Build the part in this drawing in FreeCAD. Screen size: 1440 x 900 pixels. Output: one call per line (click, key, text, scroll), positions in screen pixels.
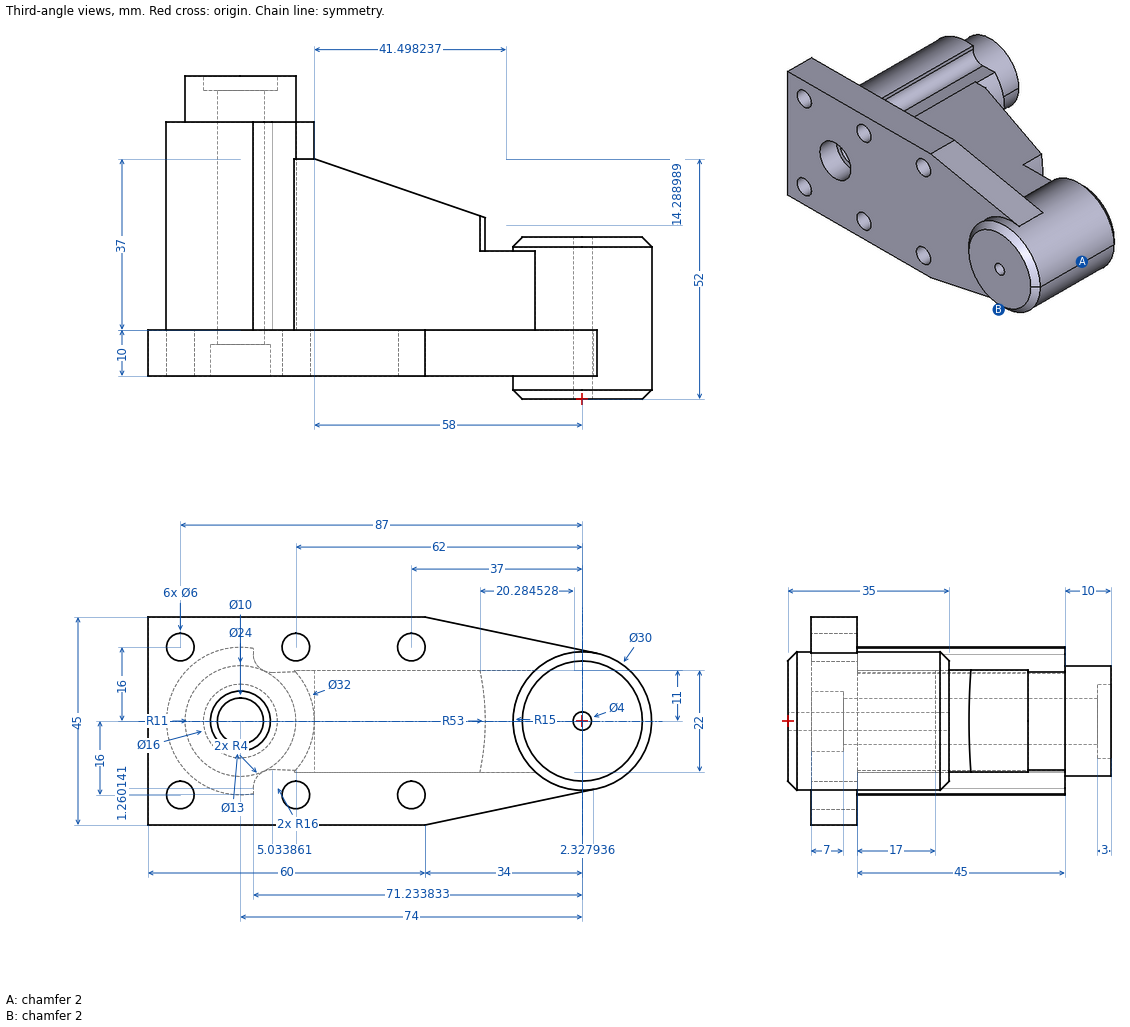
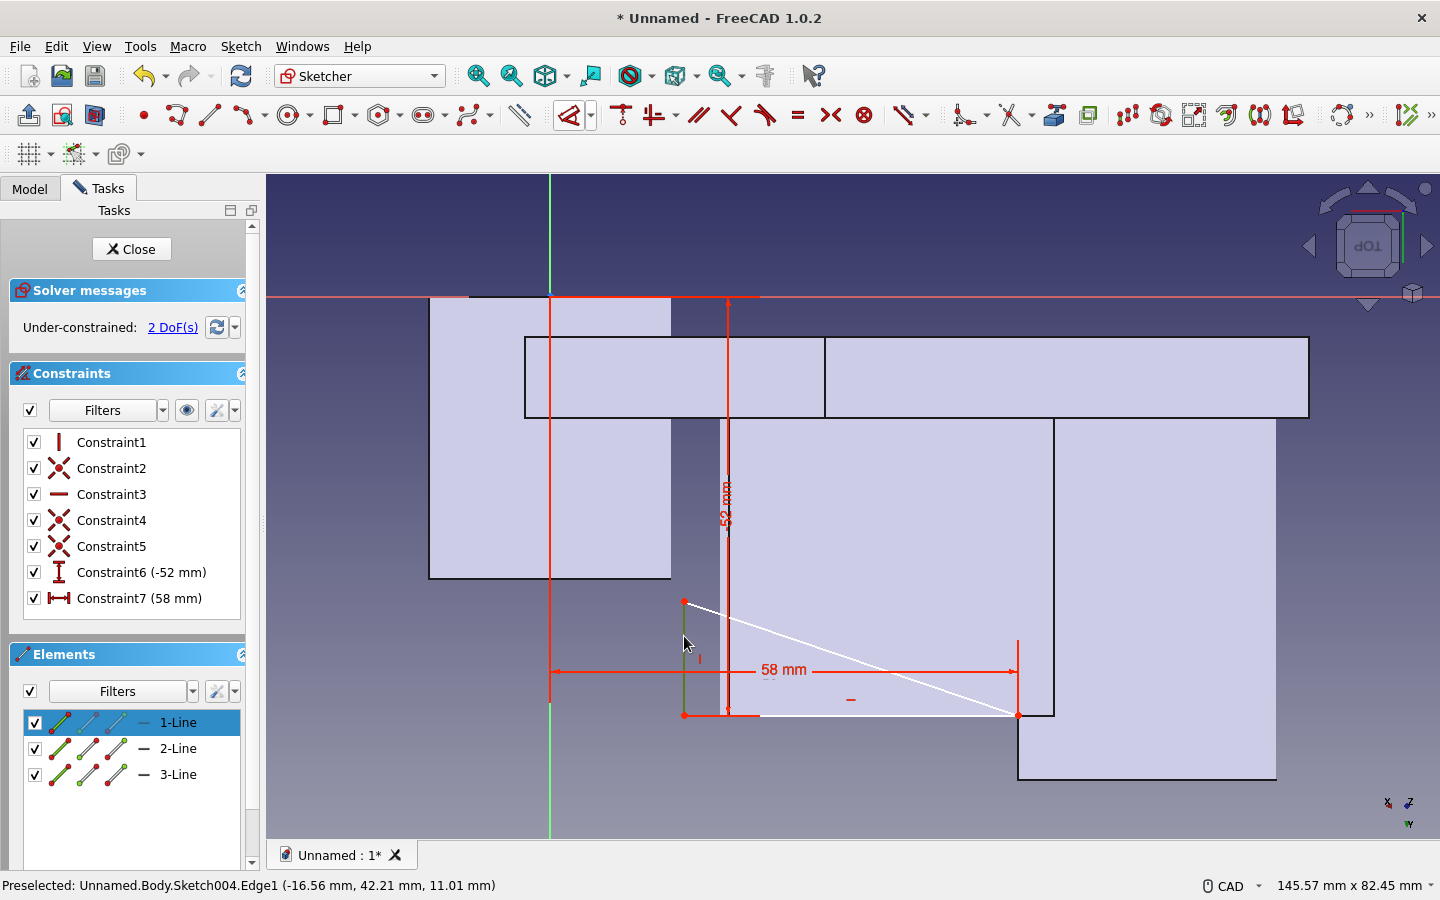
click(590, 116)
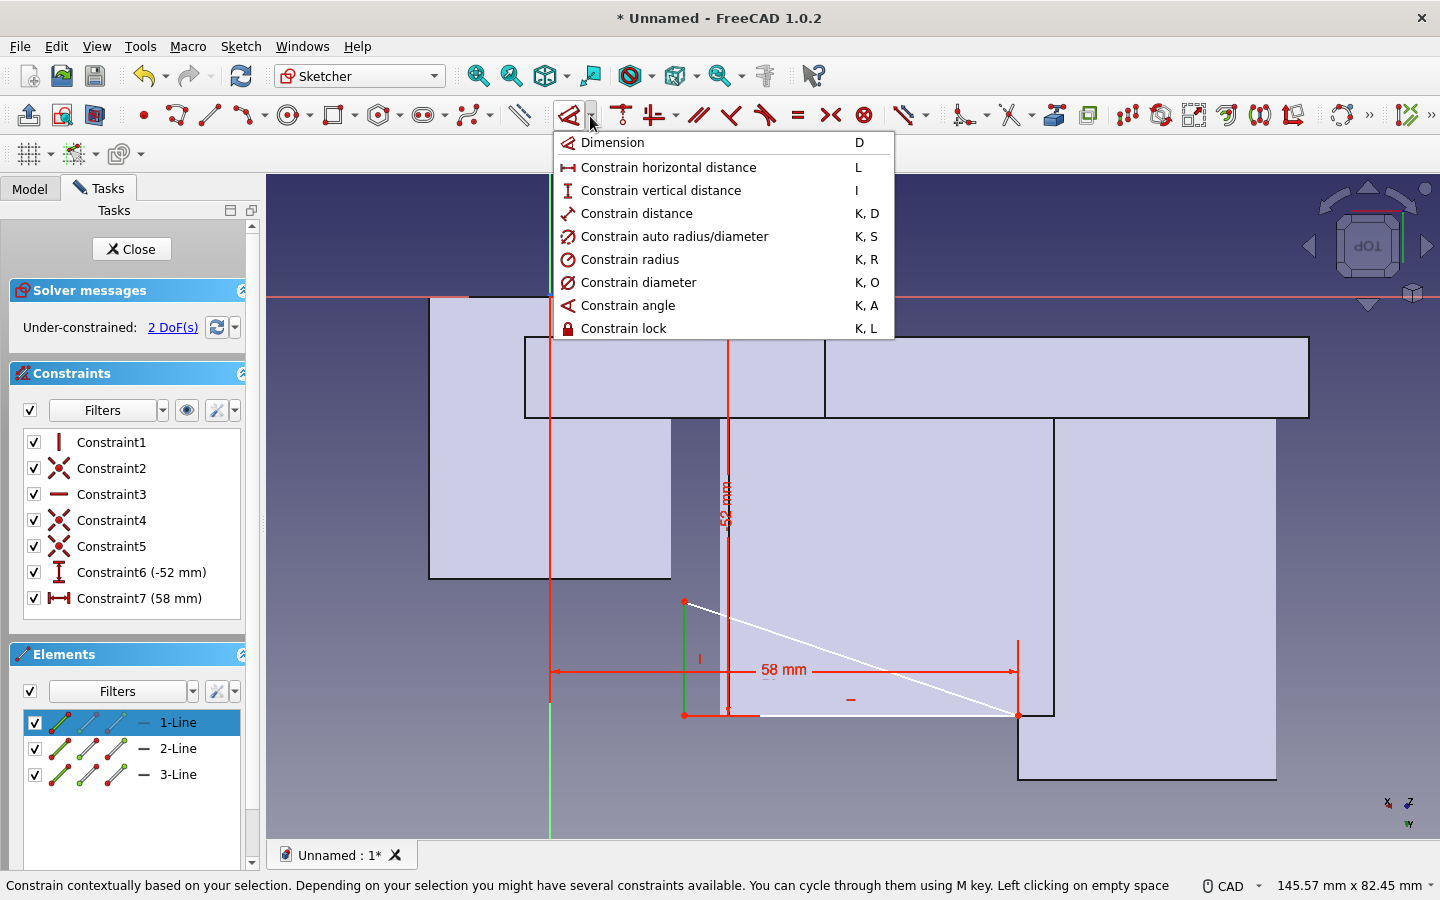
click(724, 190)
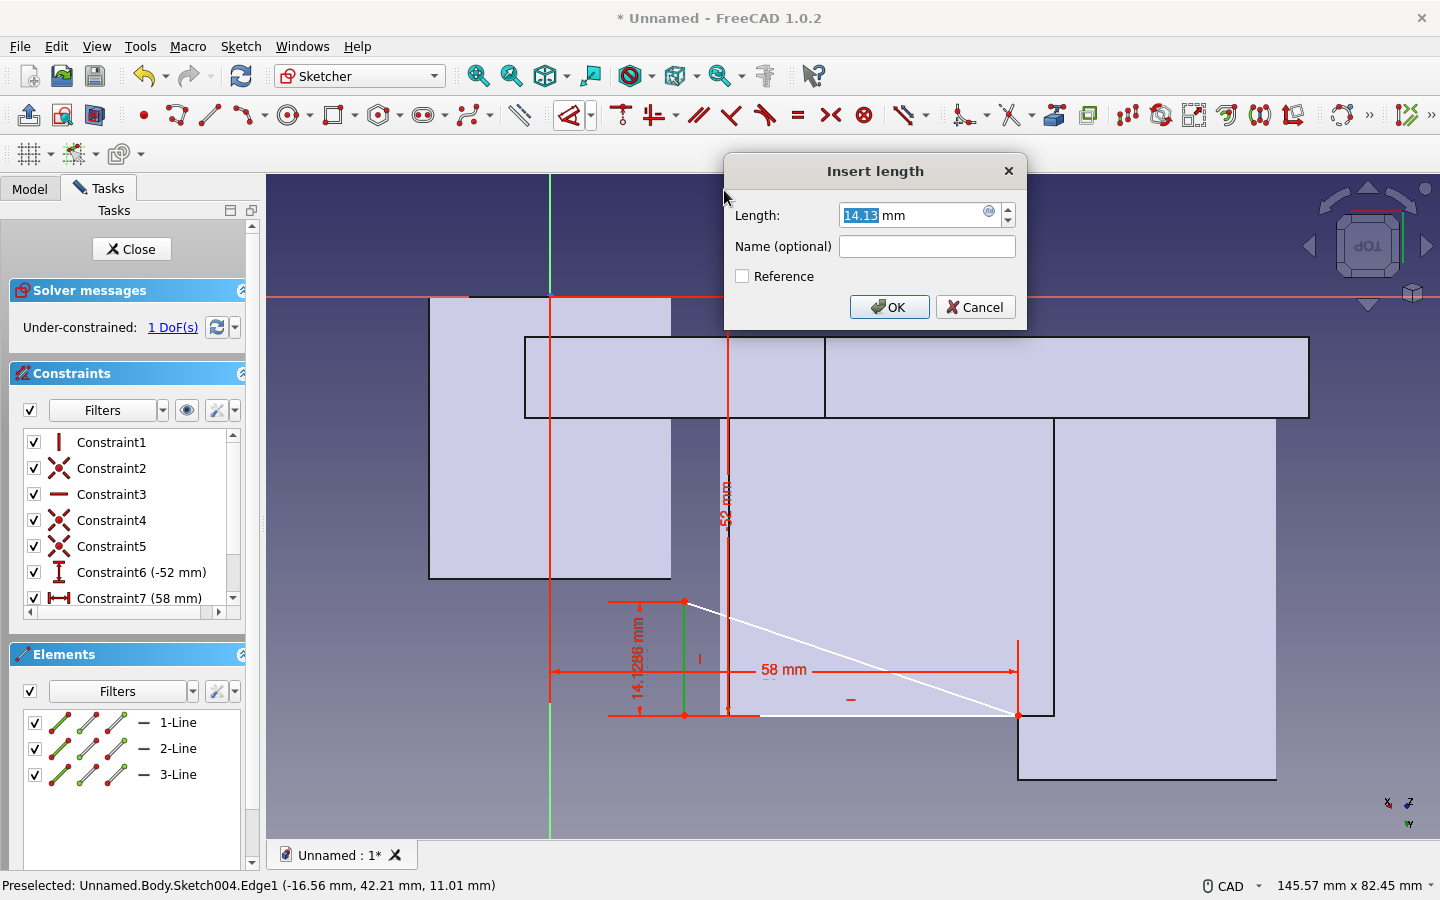
text(14.288989)
key(Return)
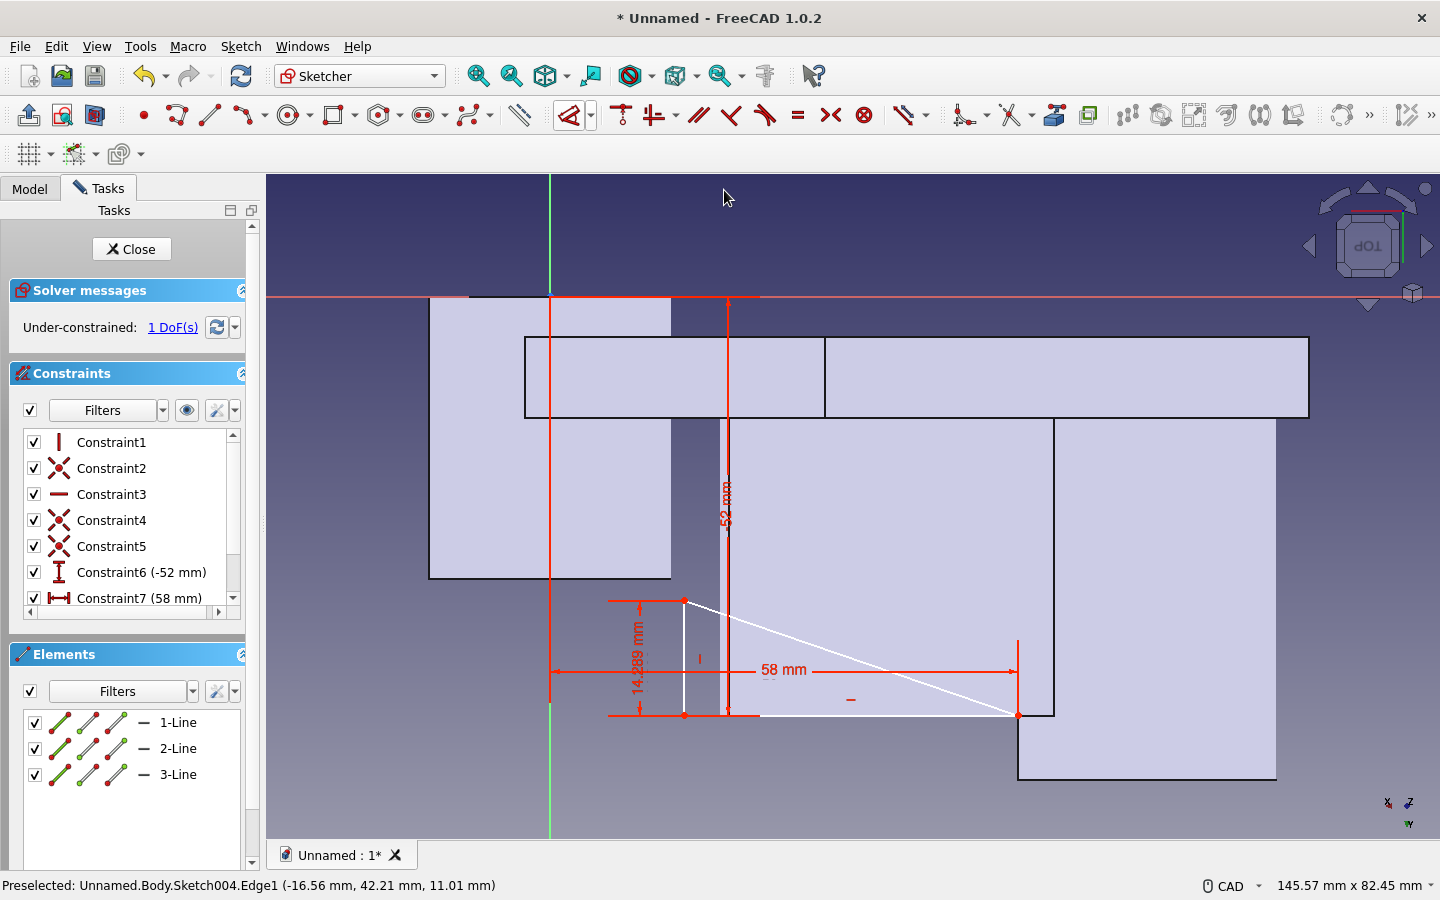
click(784, 716)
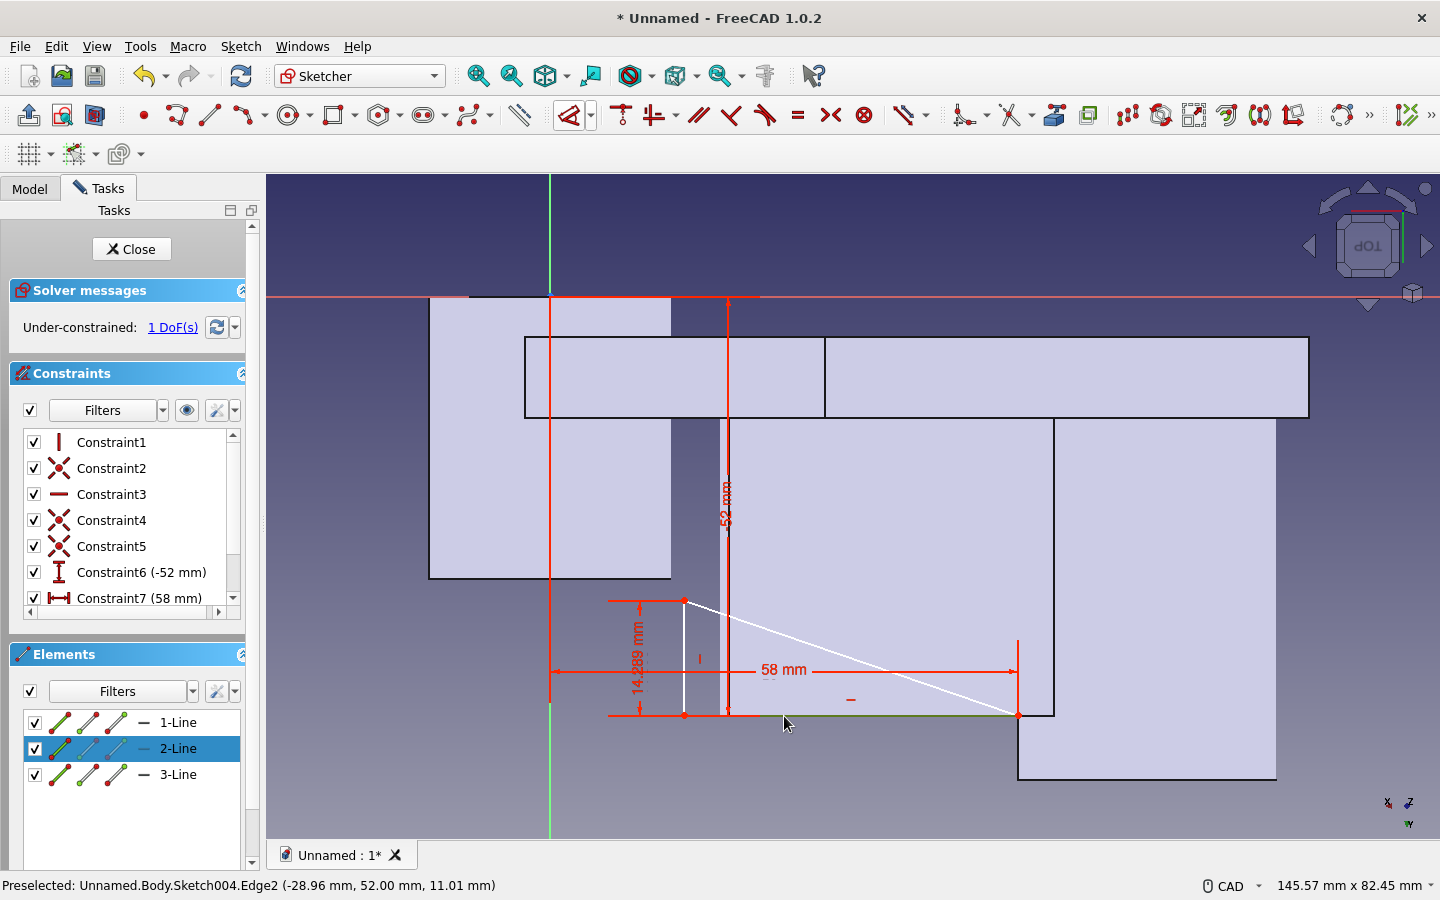
key(l)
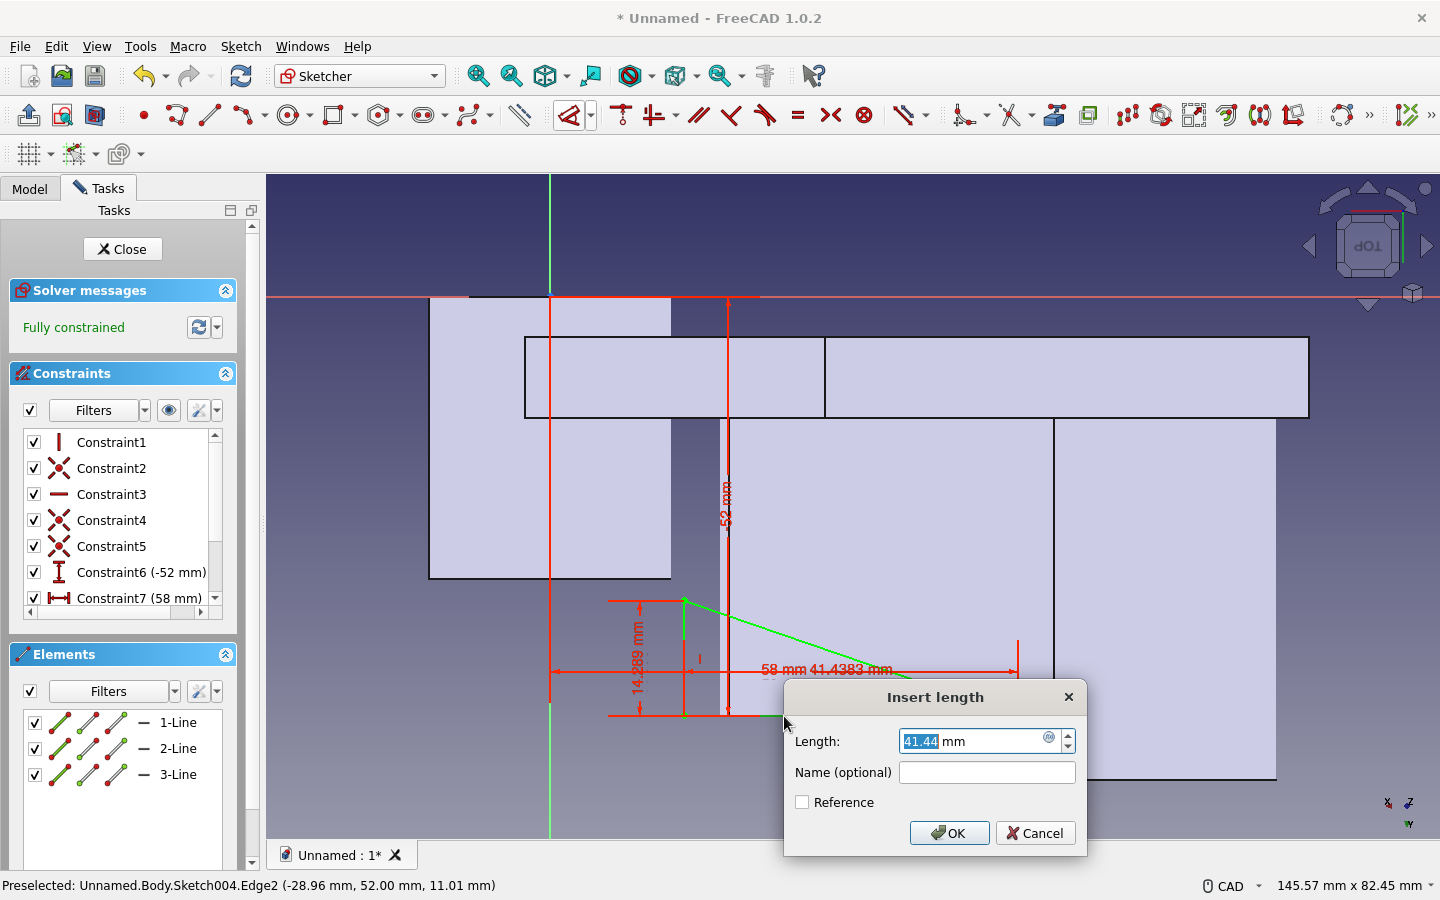
text(41.498237)
key(Return)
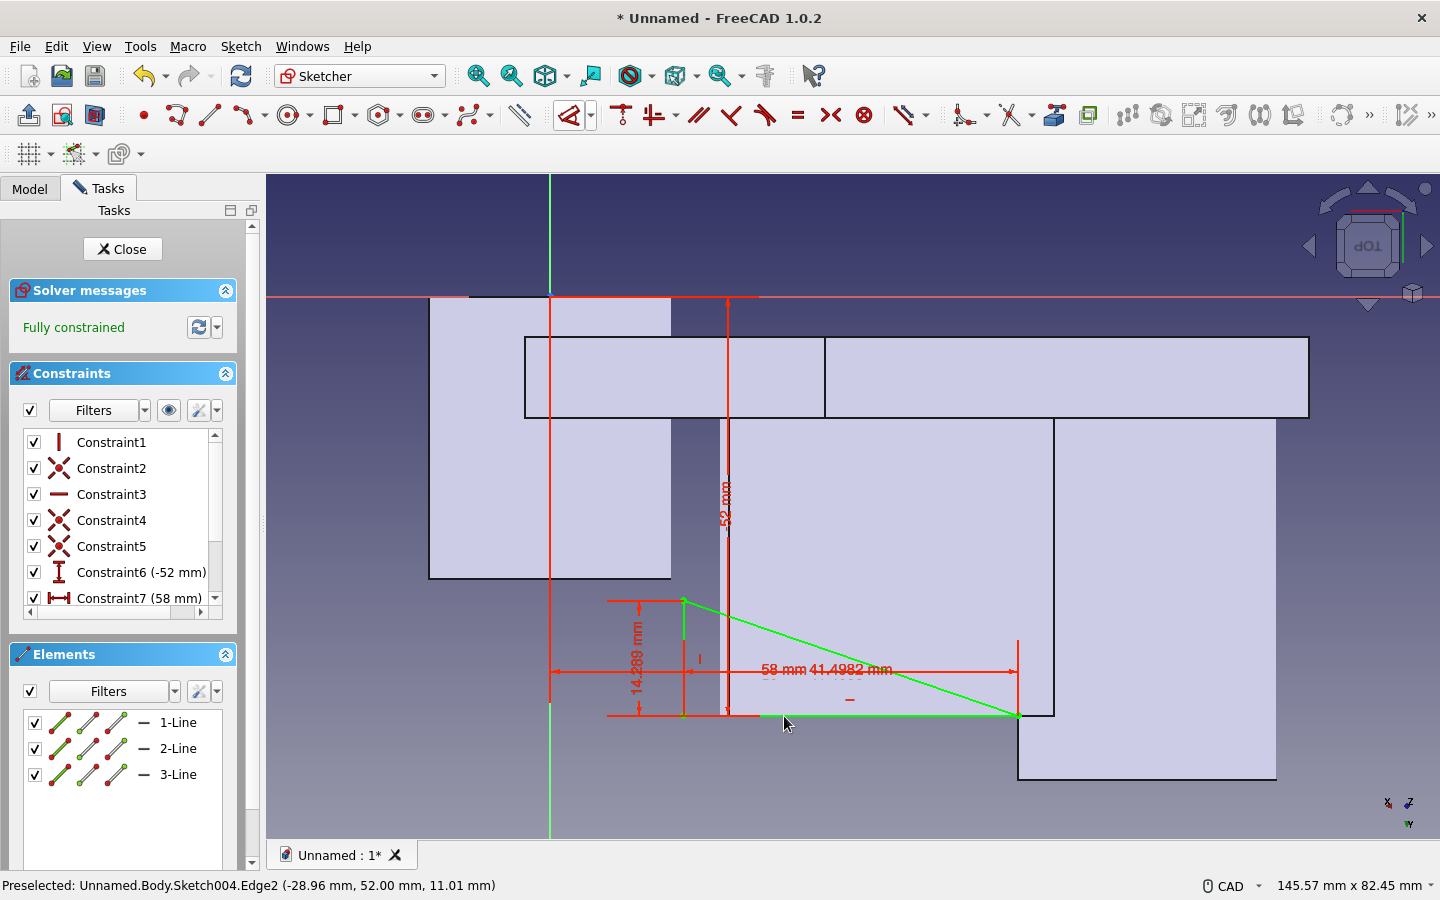
click(123, 249)